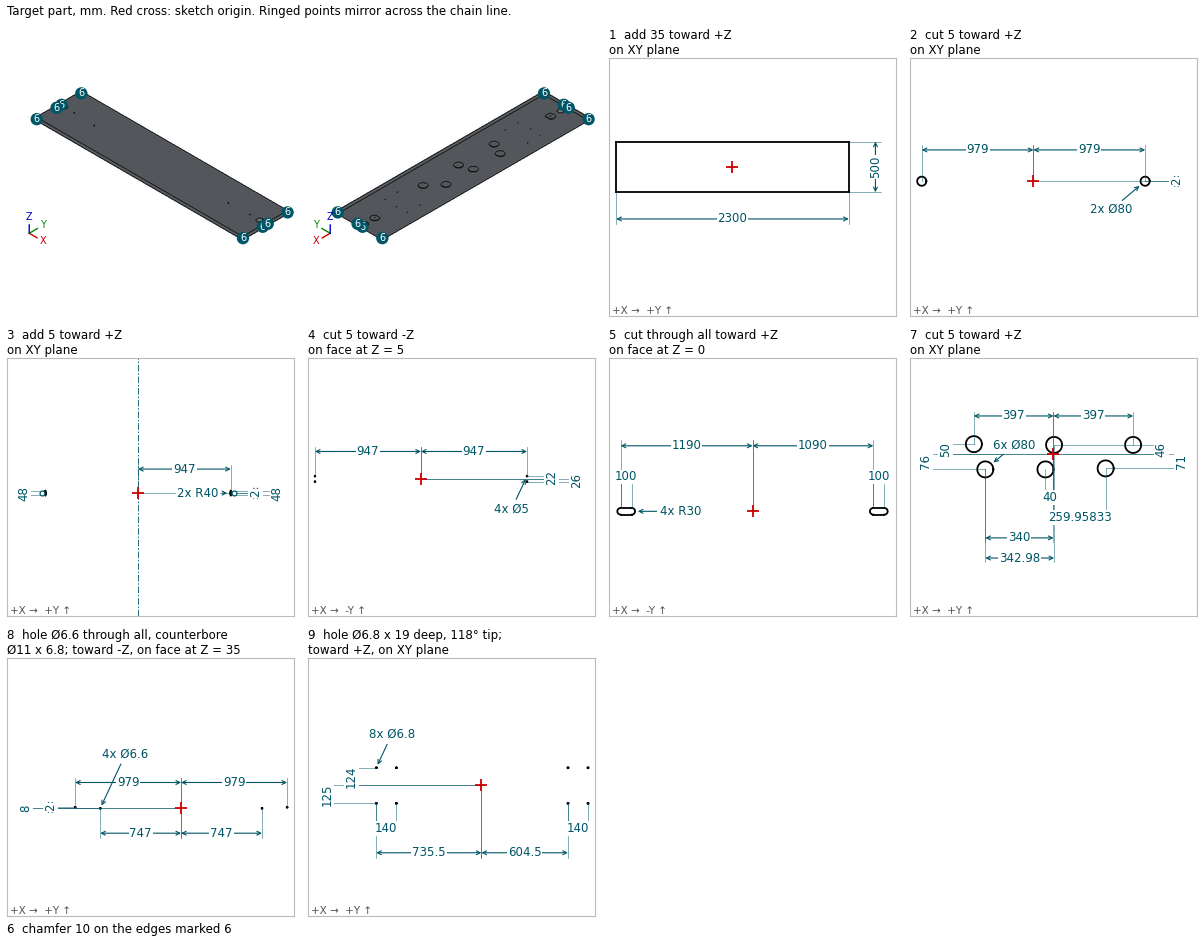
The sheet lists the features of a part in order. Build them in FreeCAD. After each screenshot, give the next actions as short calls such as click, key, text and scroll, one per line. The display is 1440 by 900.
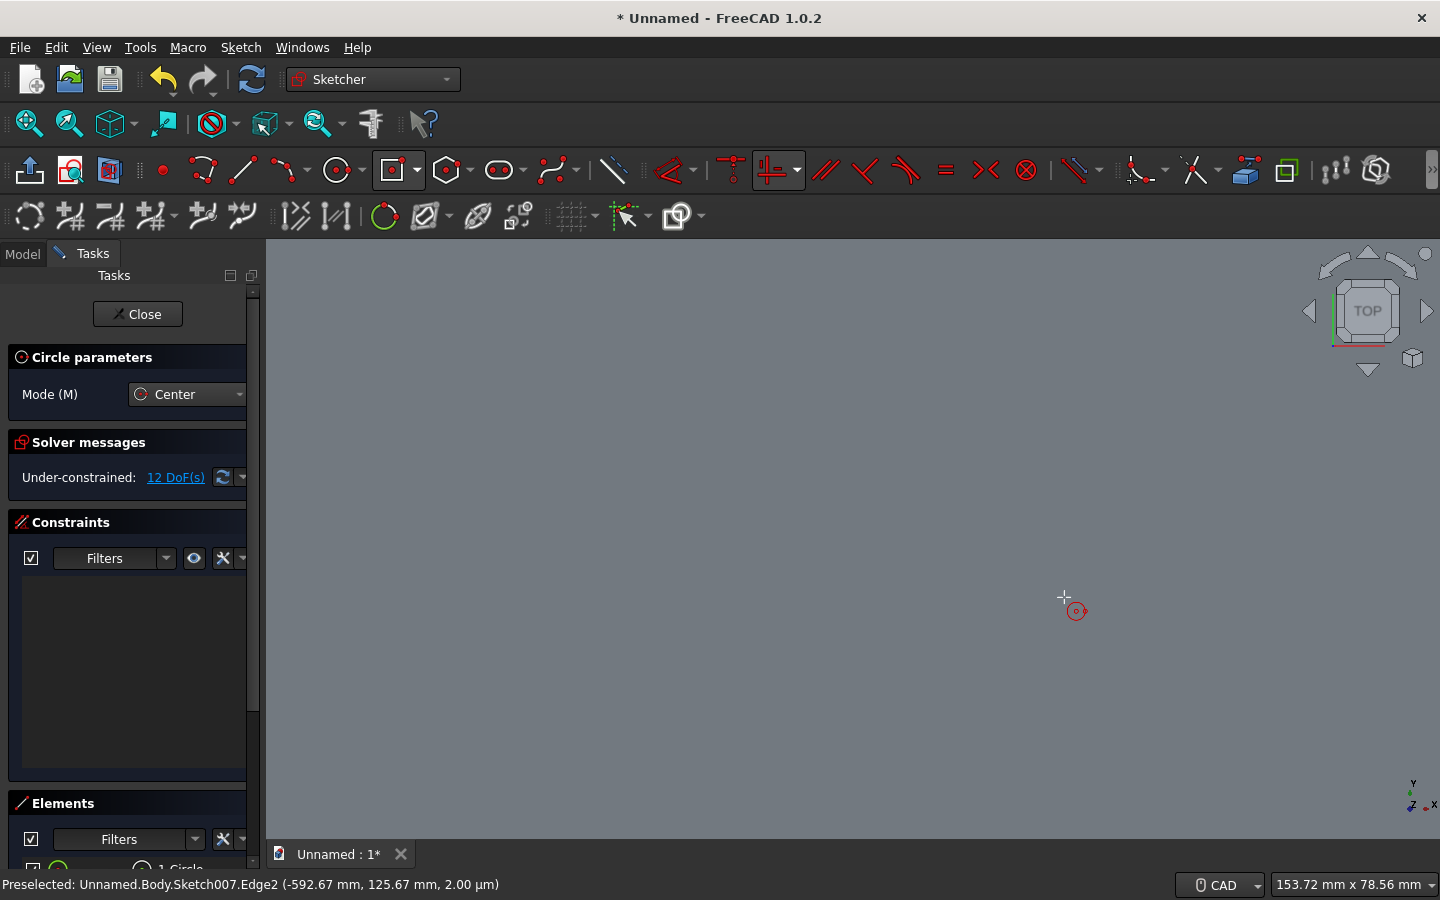
scroll(1064, 598, down, 14)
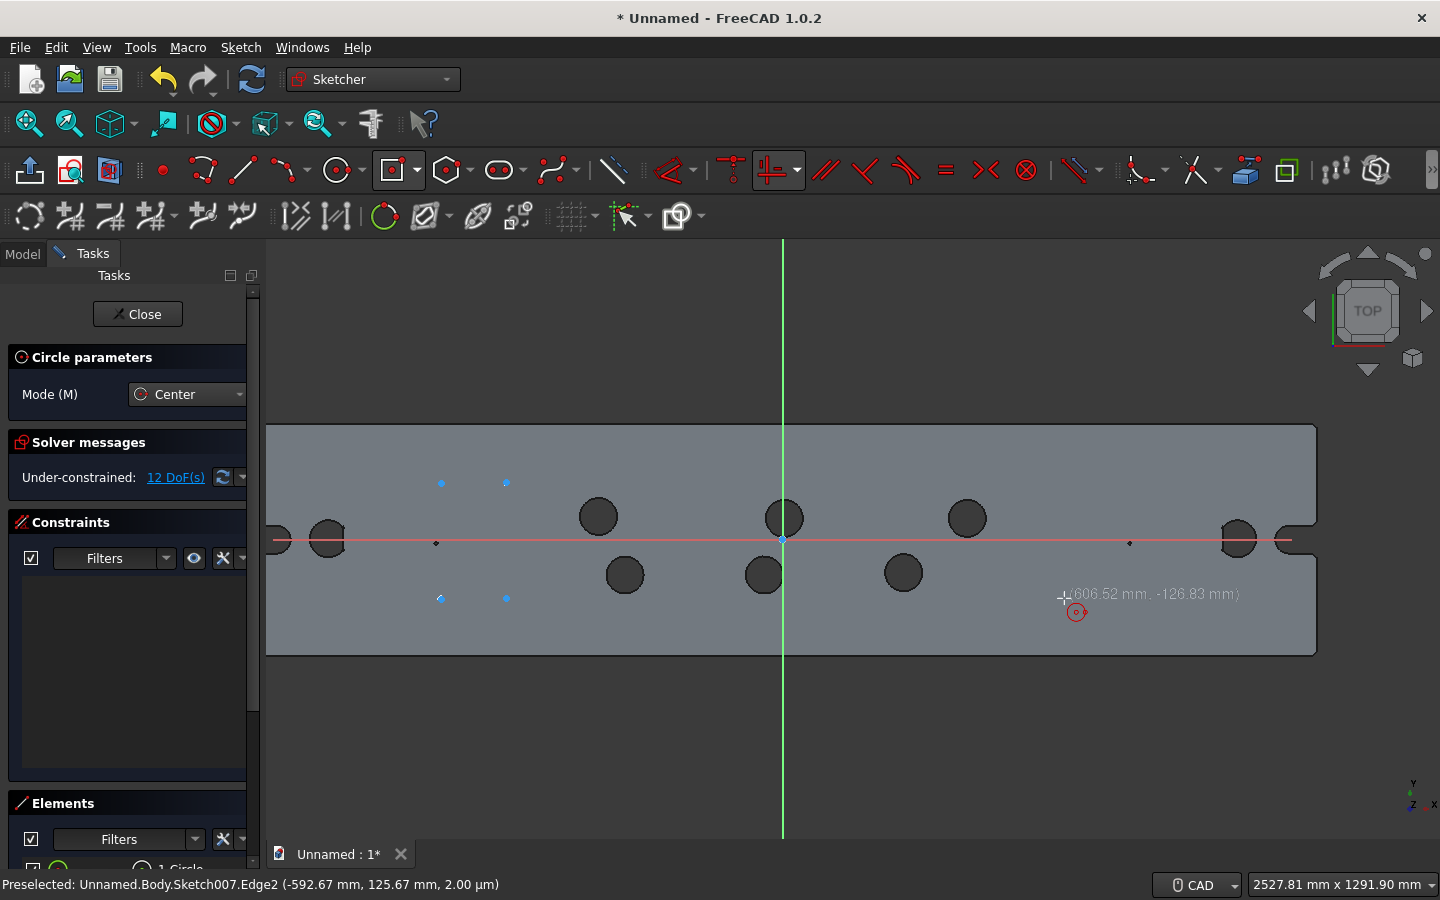
click(1064, 598)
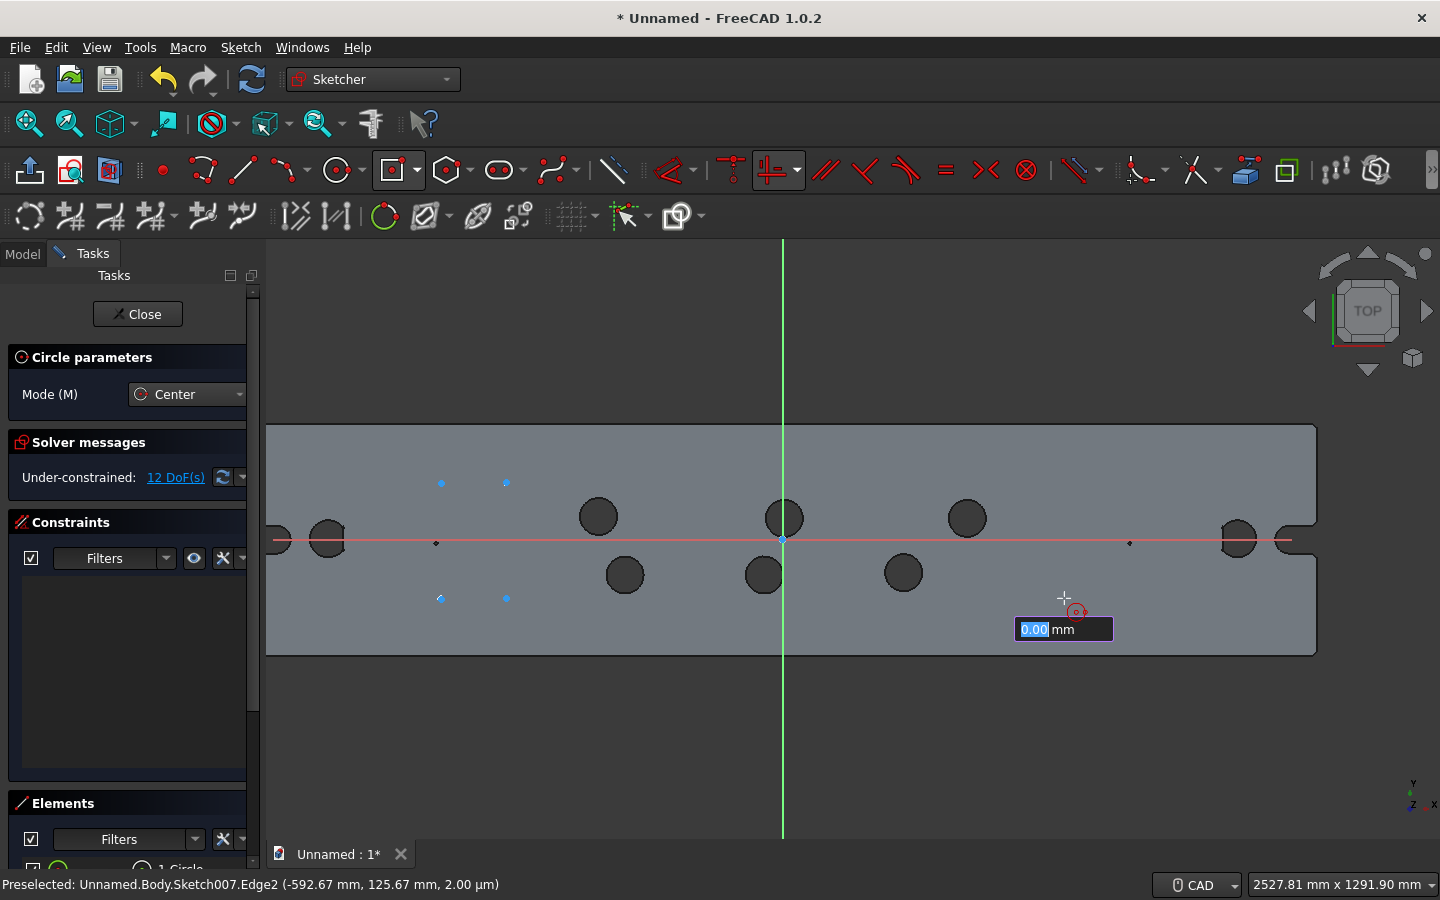
scroll(1065, 597, up, 12)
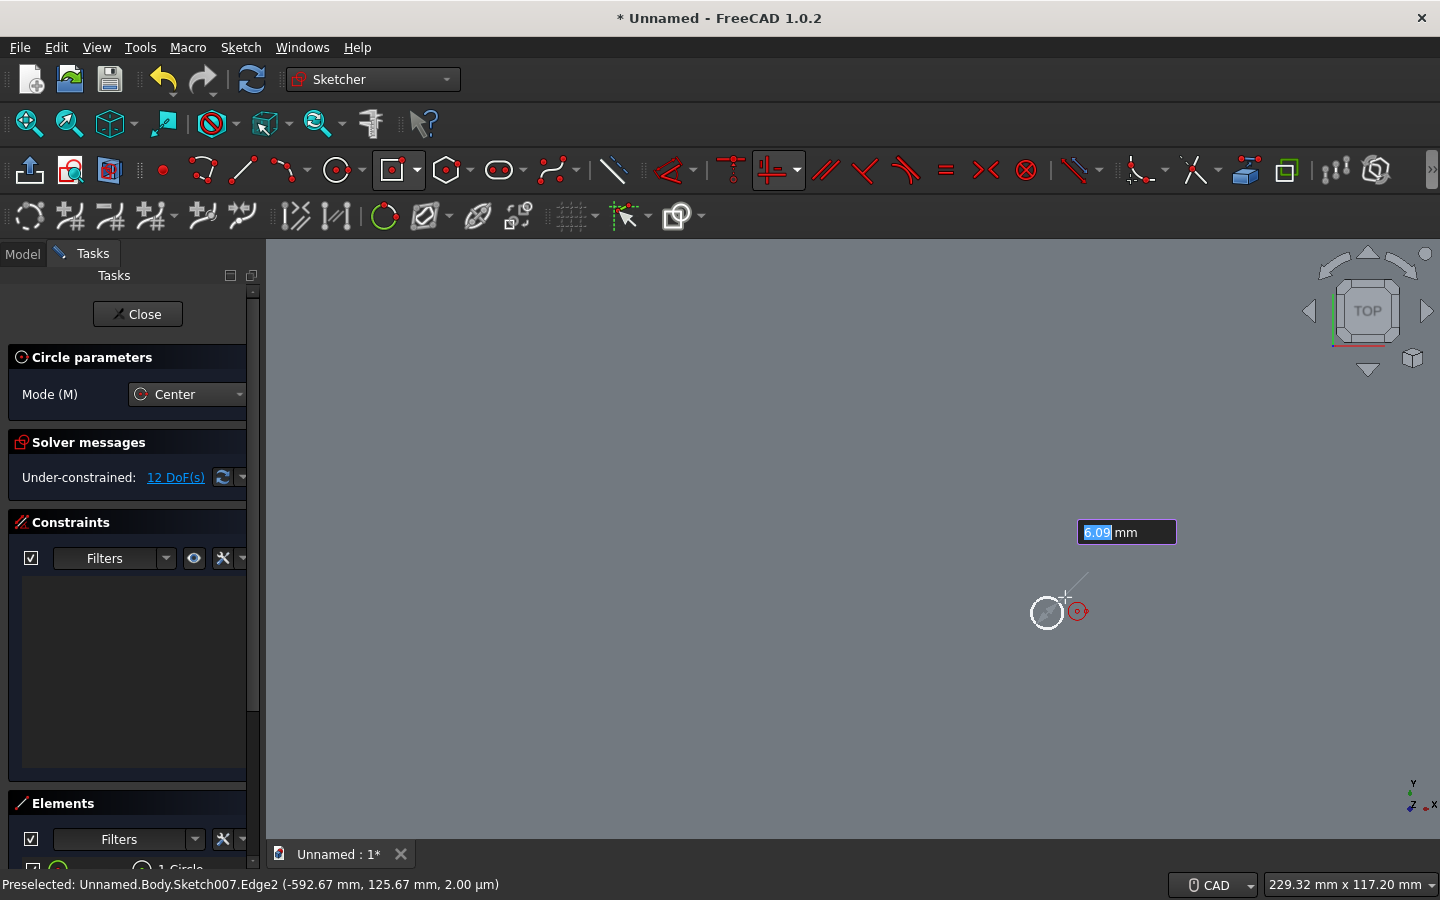
click(1056, 587)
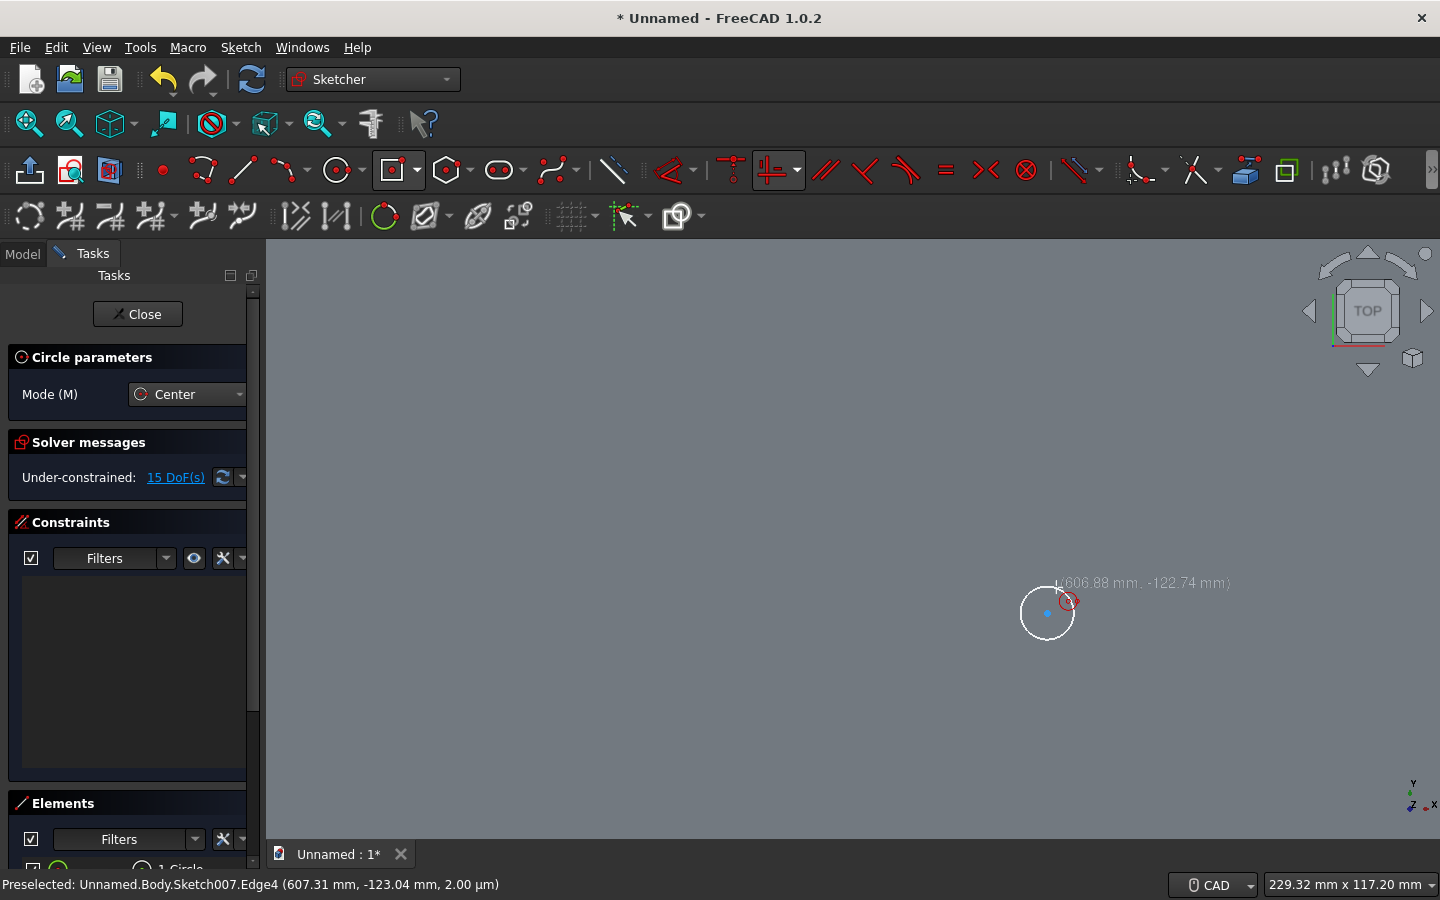
scroll(1065, 597, down, 12)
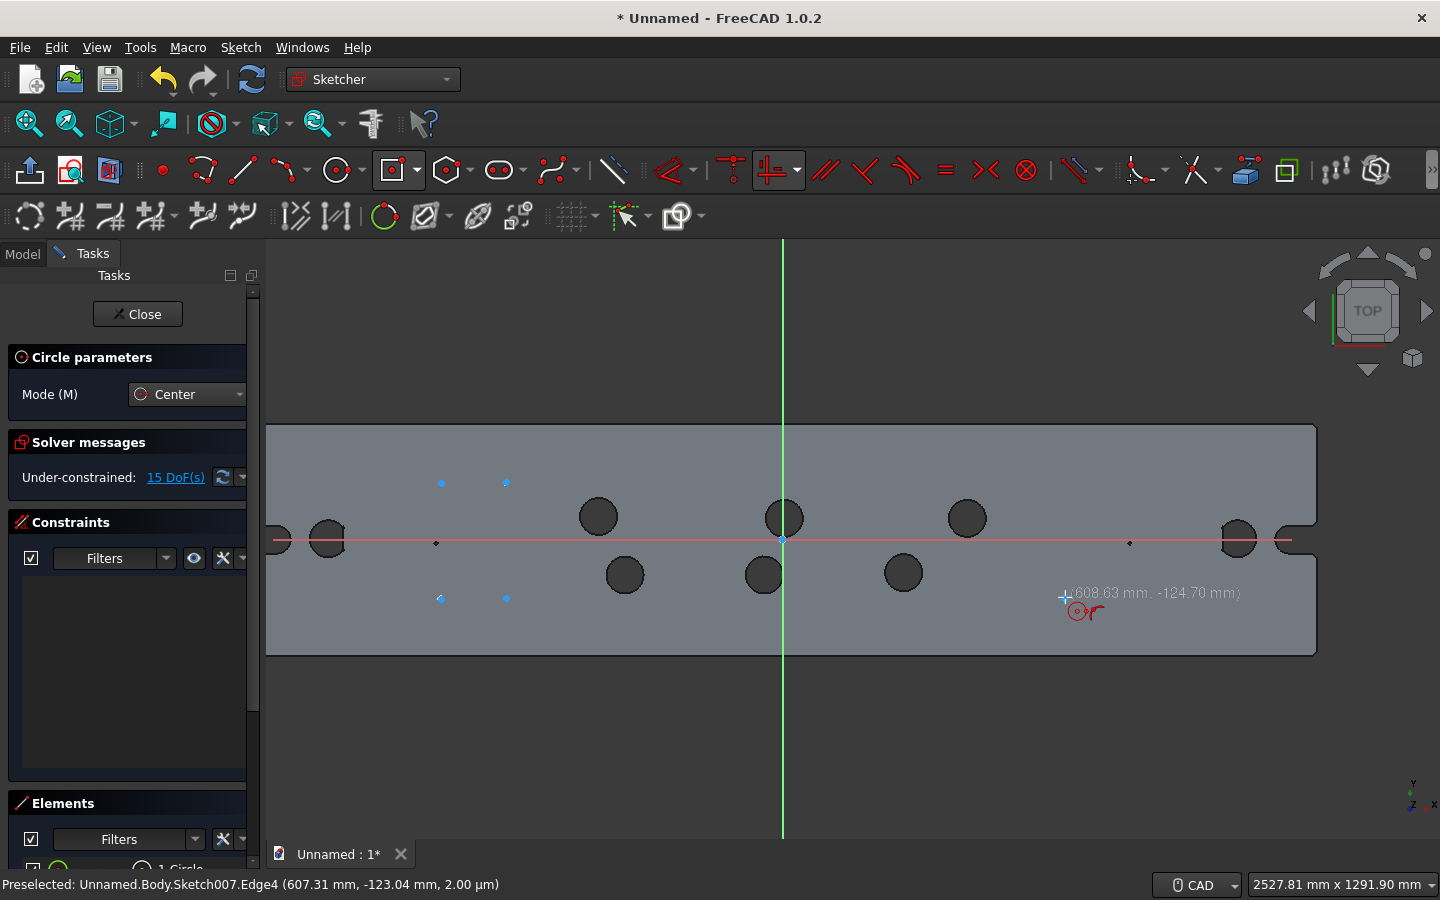
scroll(1129, 598, up, 14)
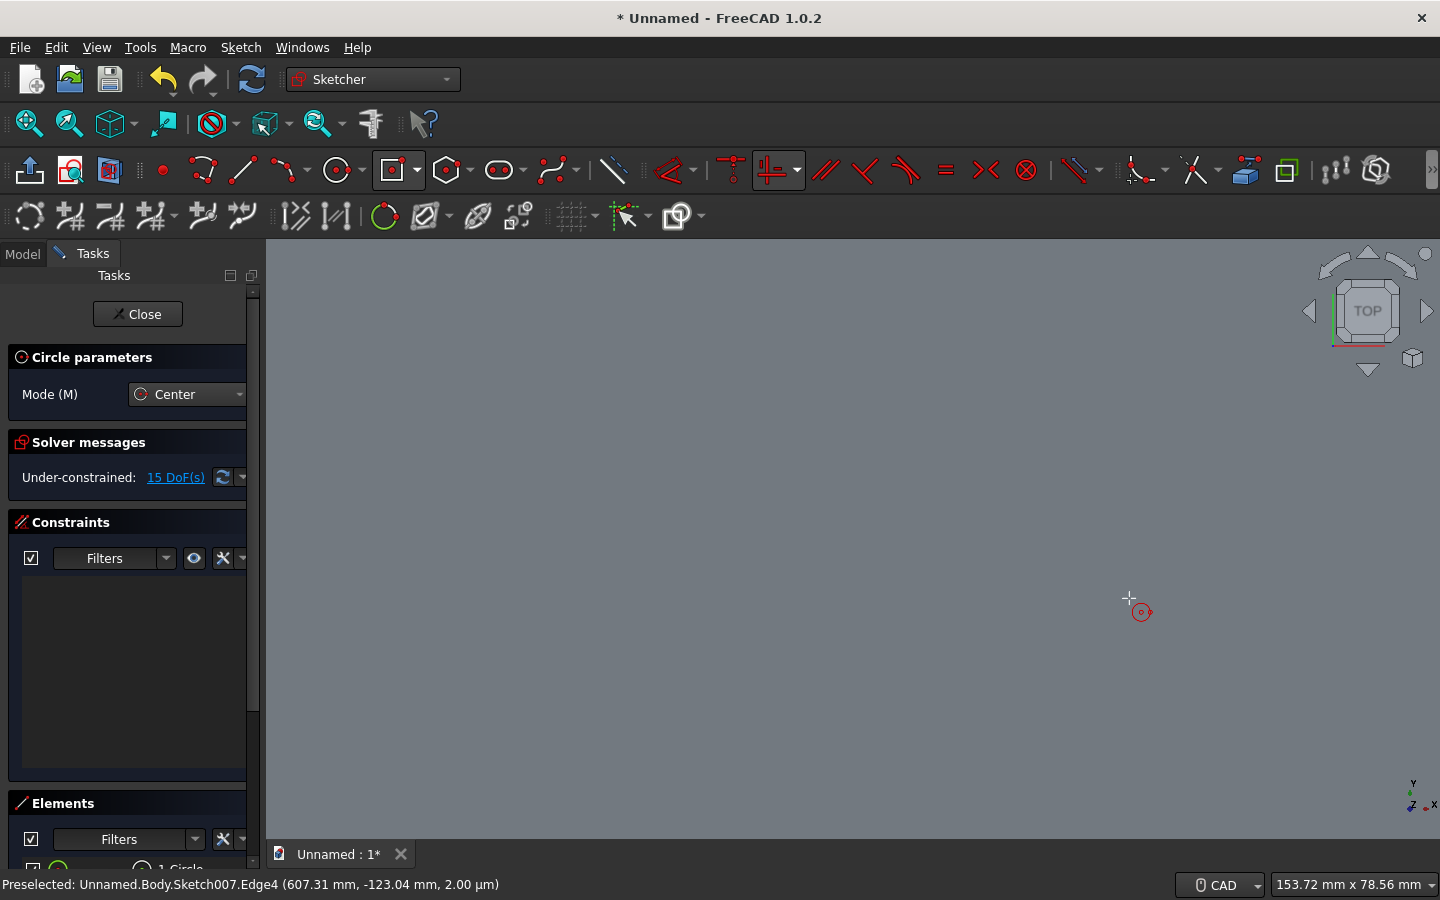
scroll(1129, 598, down, 14)